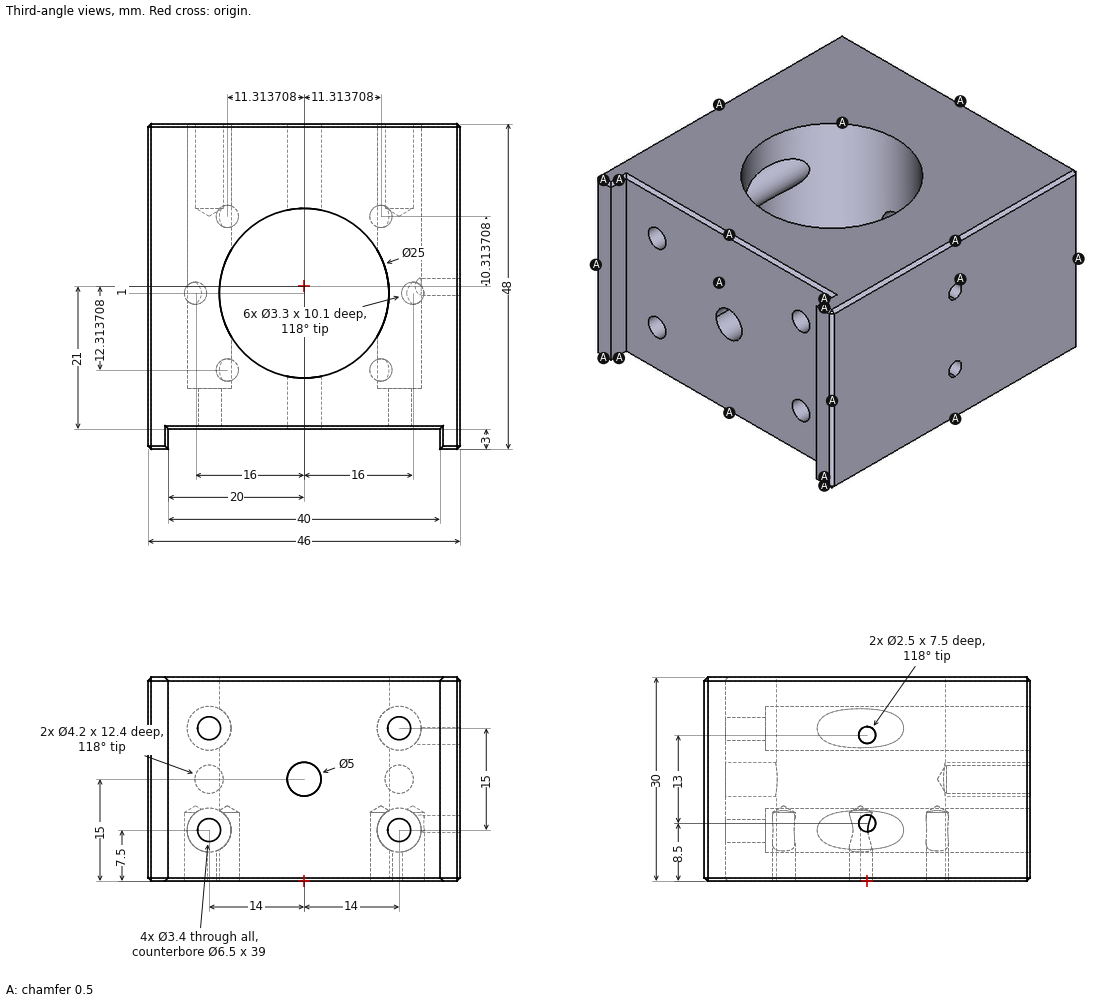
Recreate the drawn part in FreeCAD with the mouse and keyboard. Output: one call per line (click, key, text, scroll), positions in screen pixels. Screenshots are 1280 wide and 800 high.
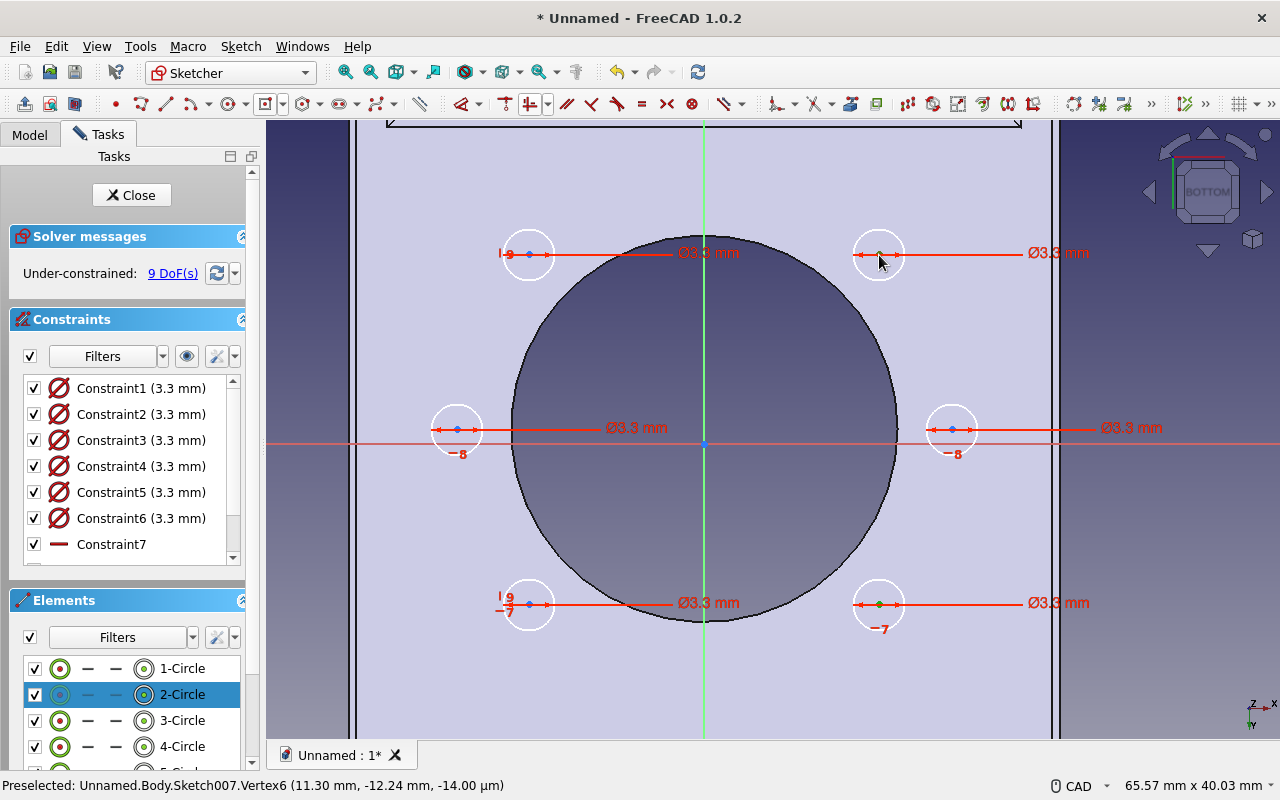
key(v)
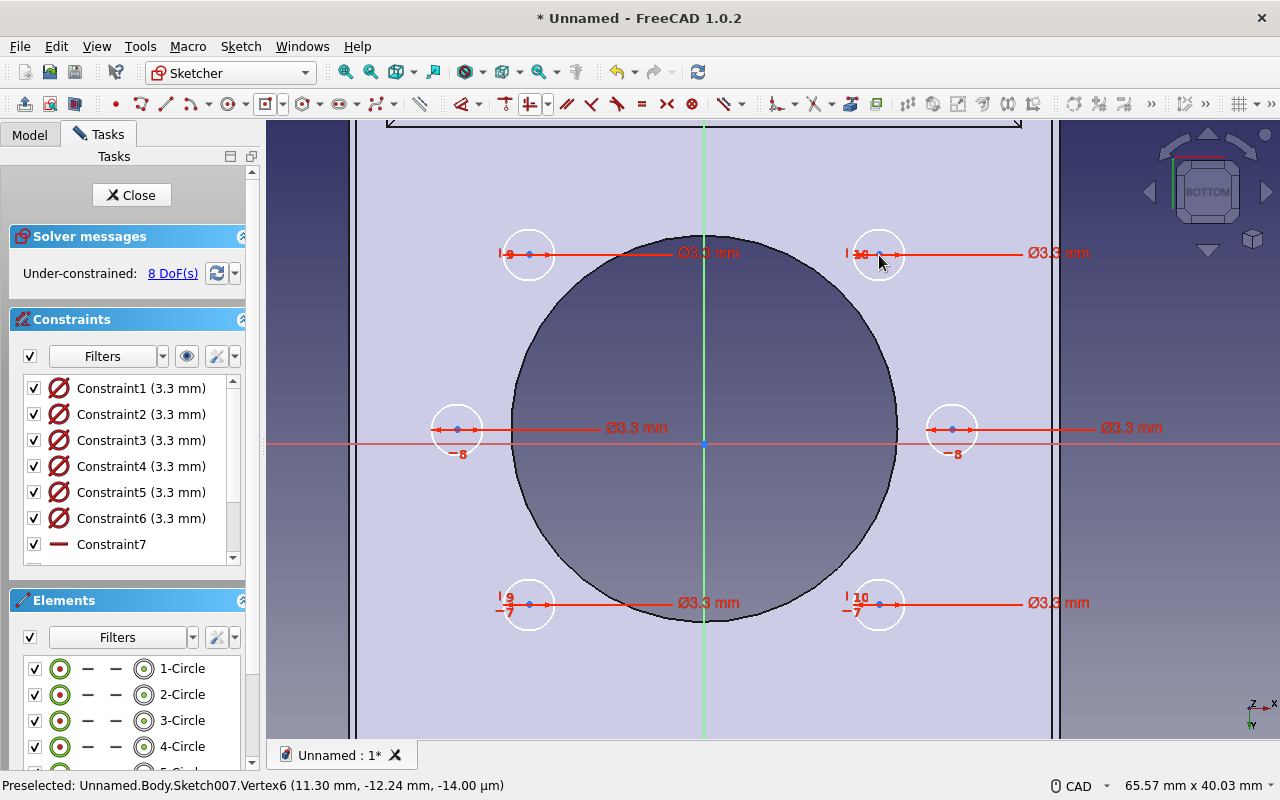
click(529, 255)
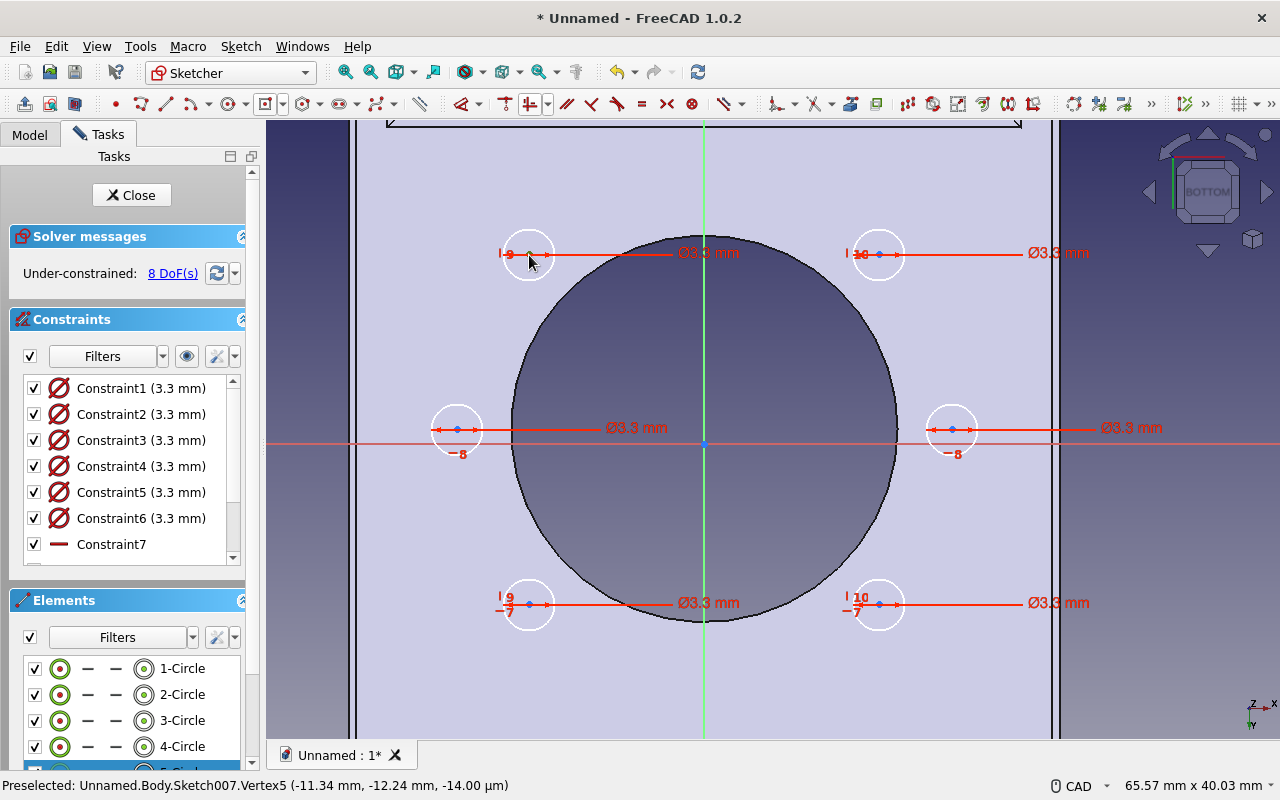
click(879, 255)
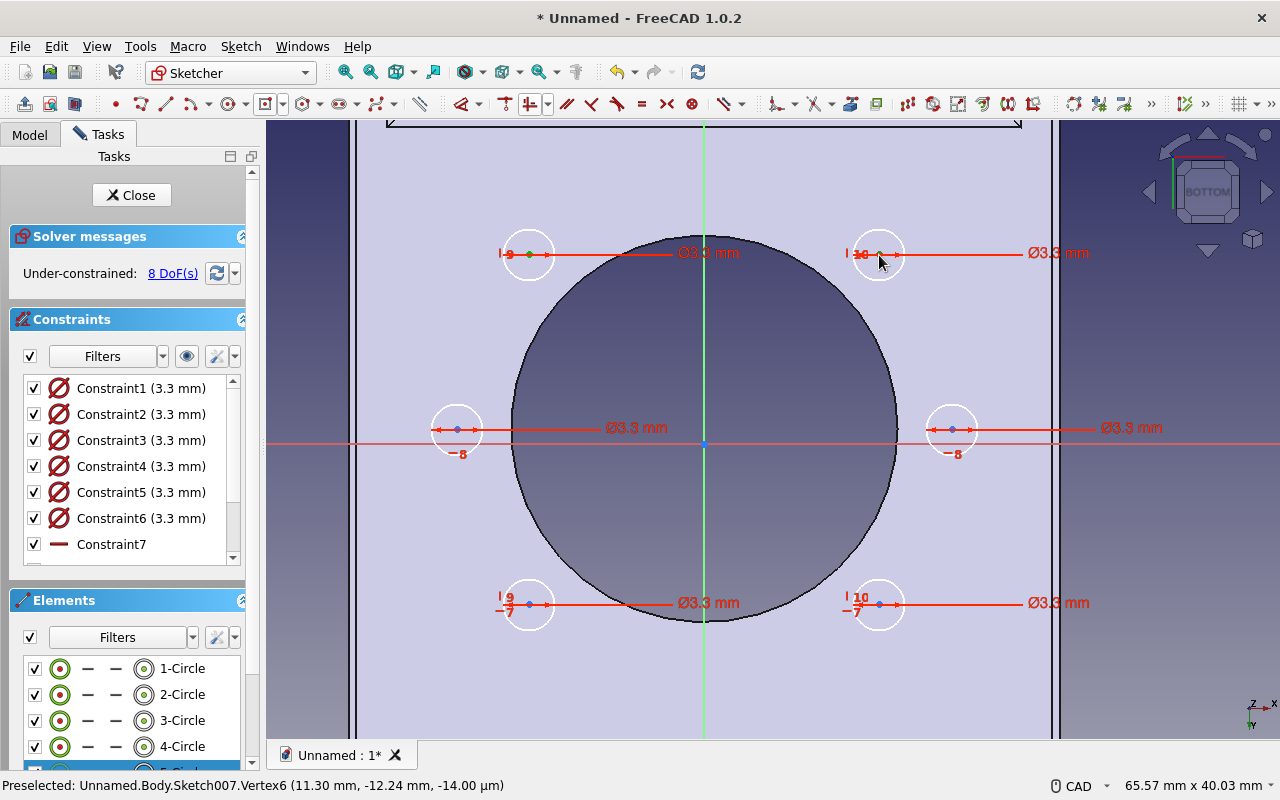
click(548, 104)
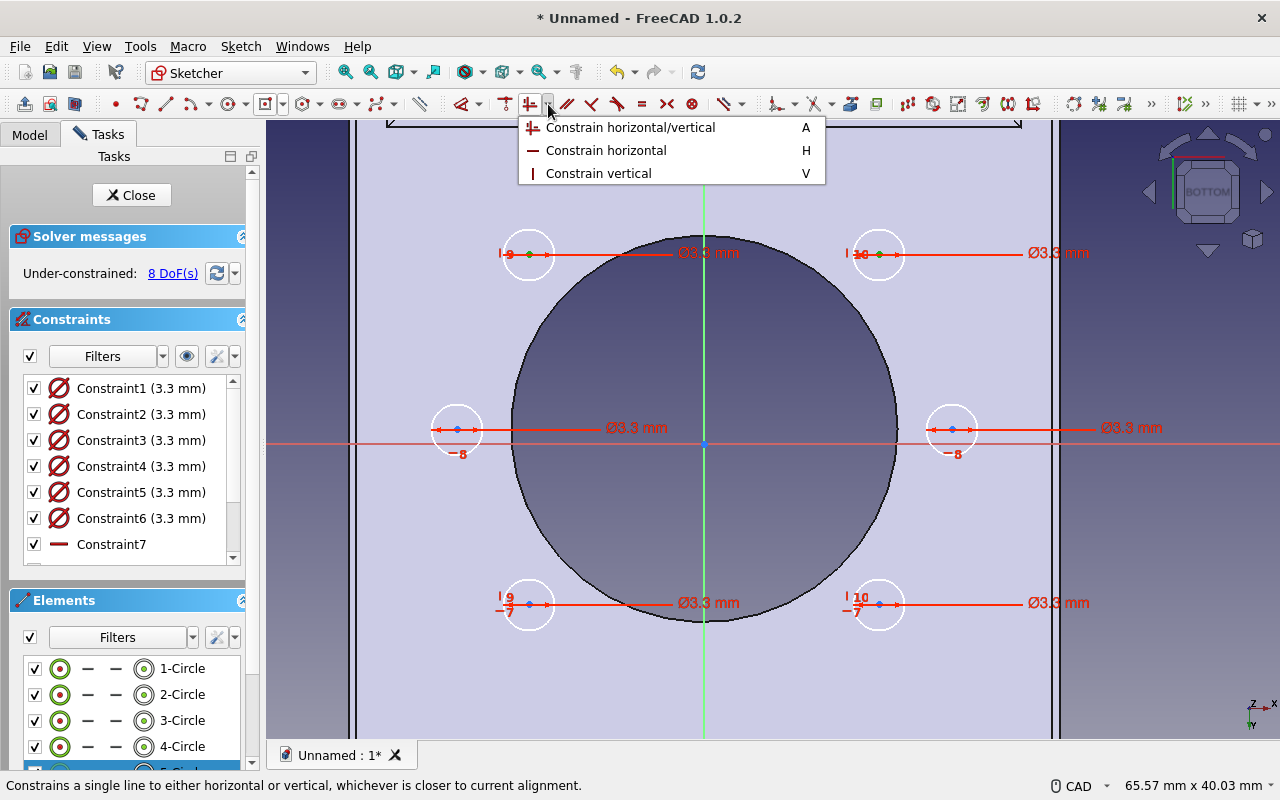
click(672, 150)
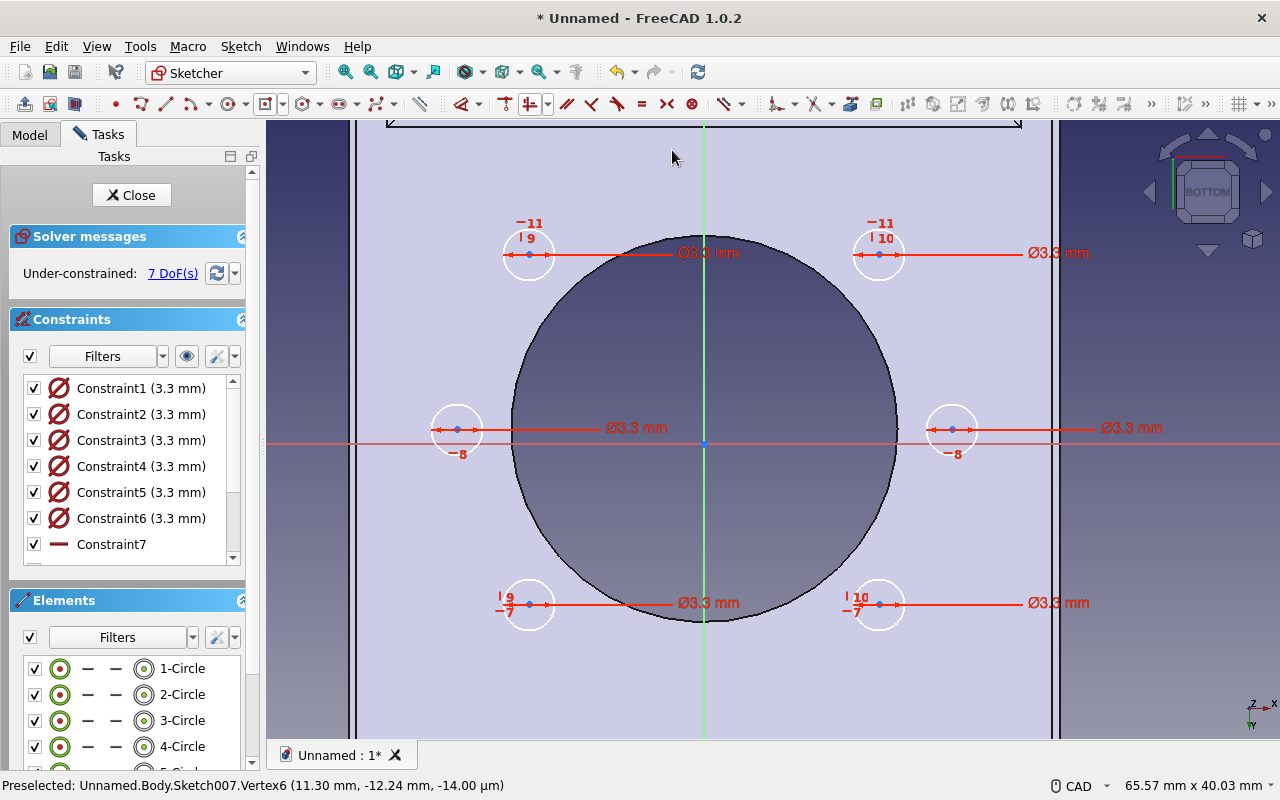
click(460, 104)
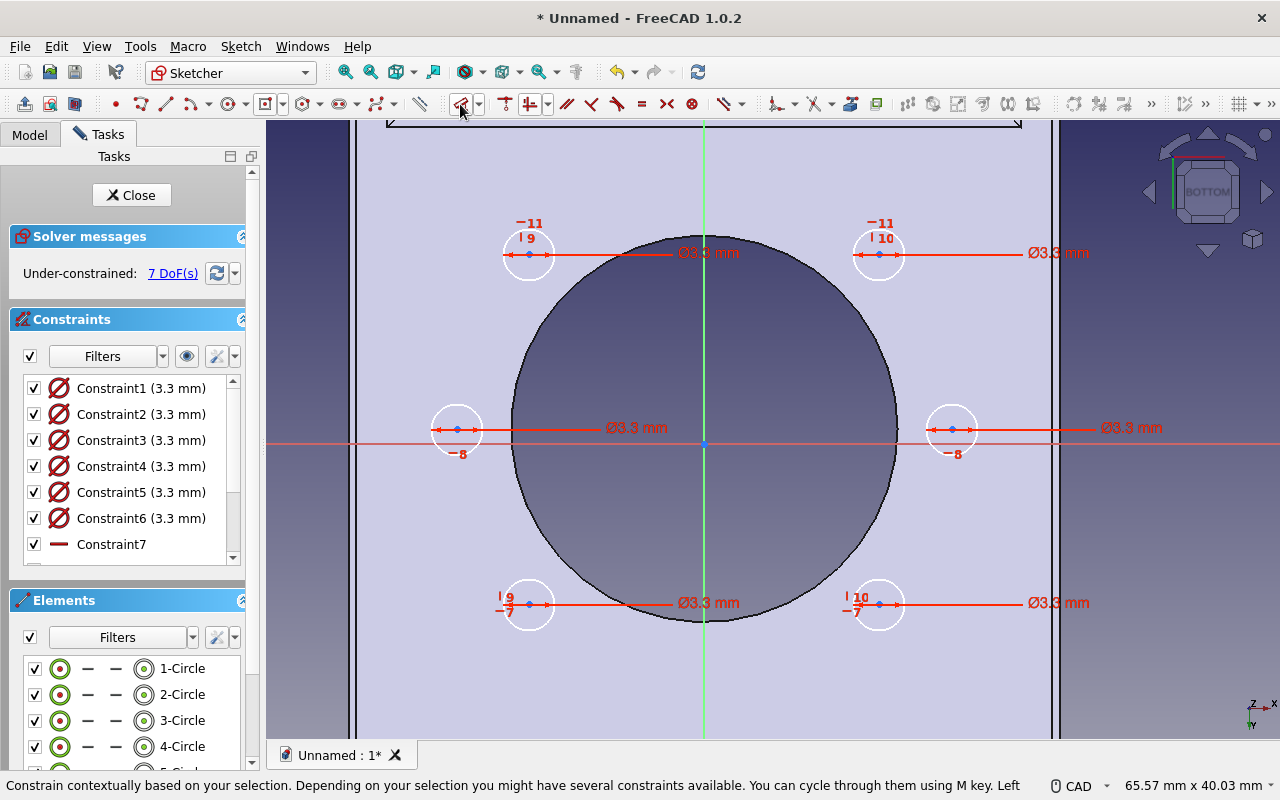
scroll(952, 430, up, 5)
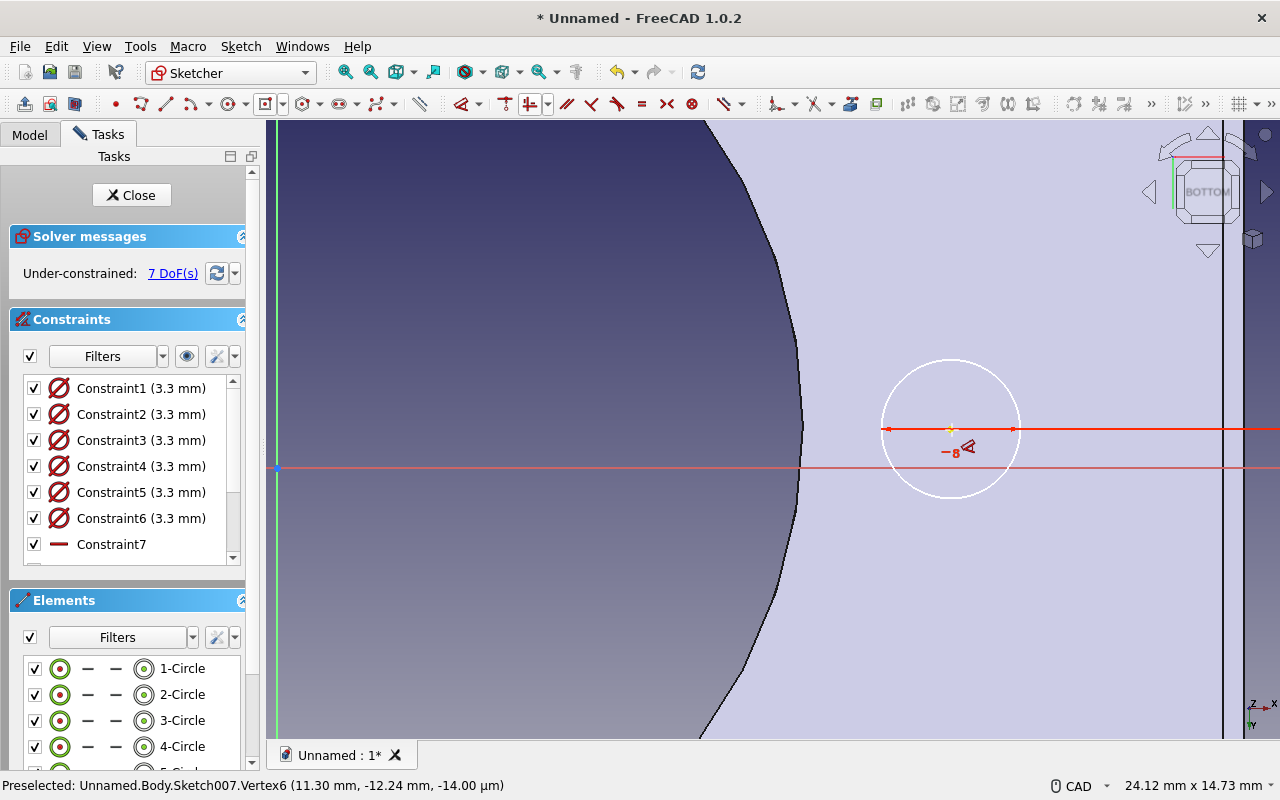
click(951, 429)
click(985, 449)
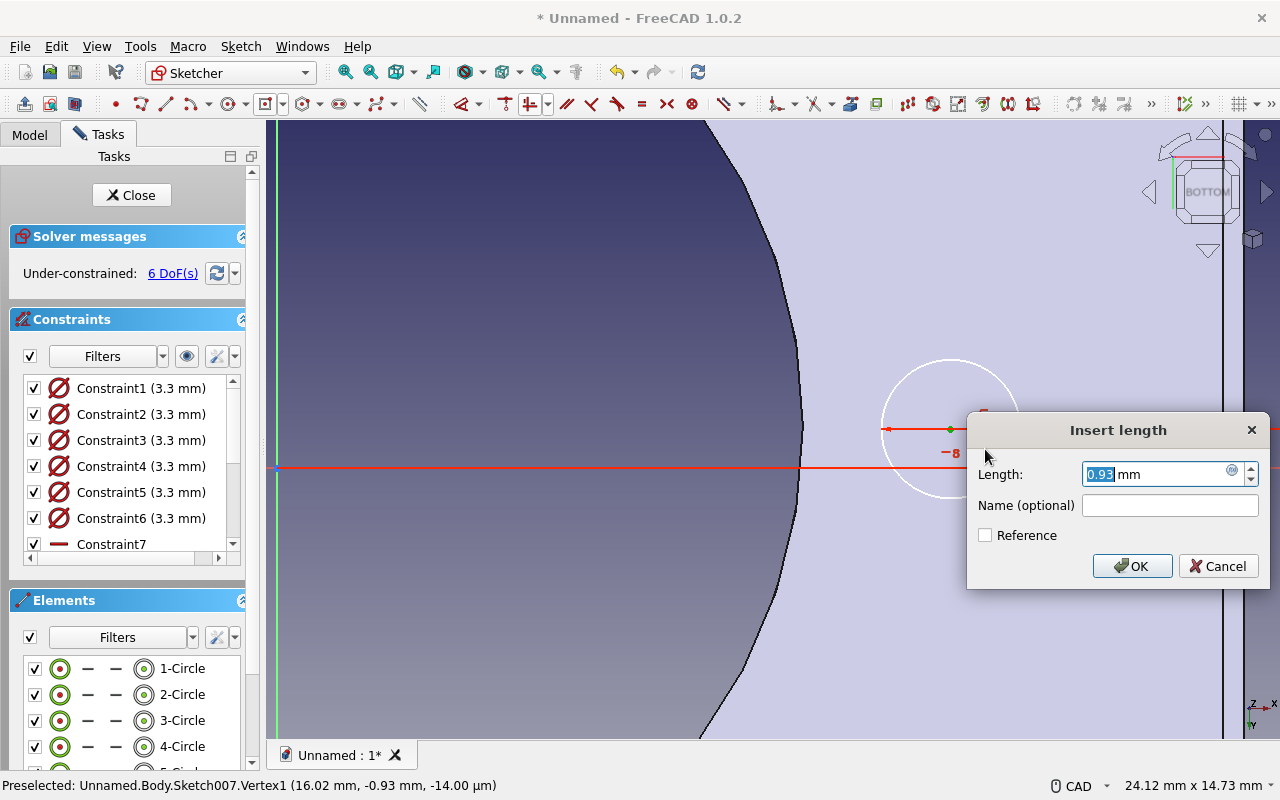
text(1)
key(Return)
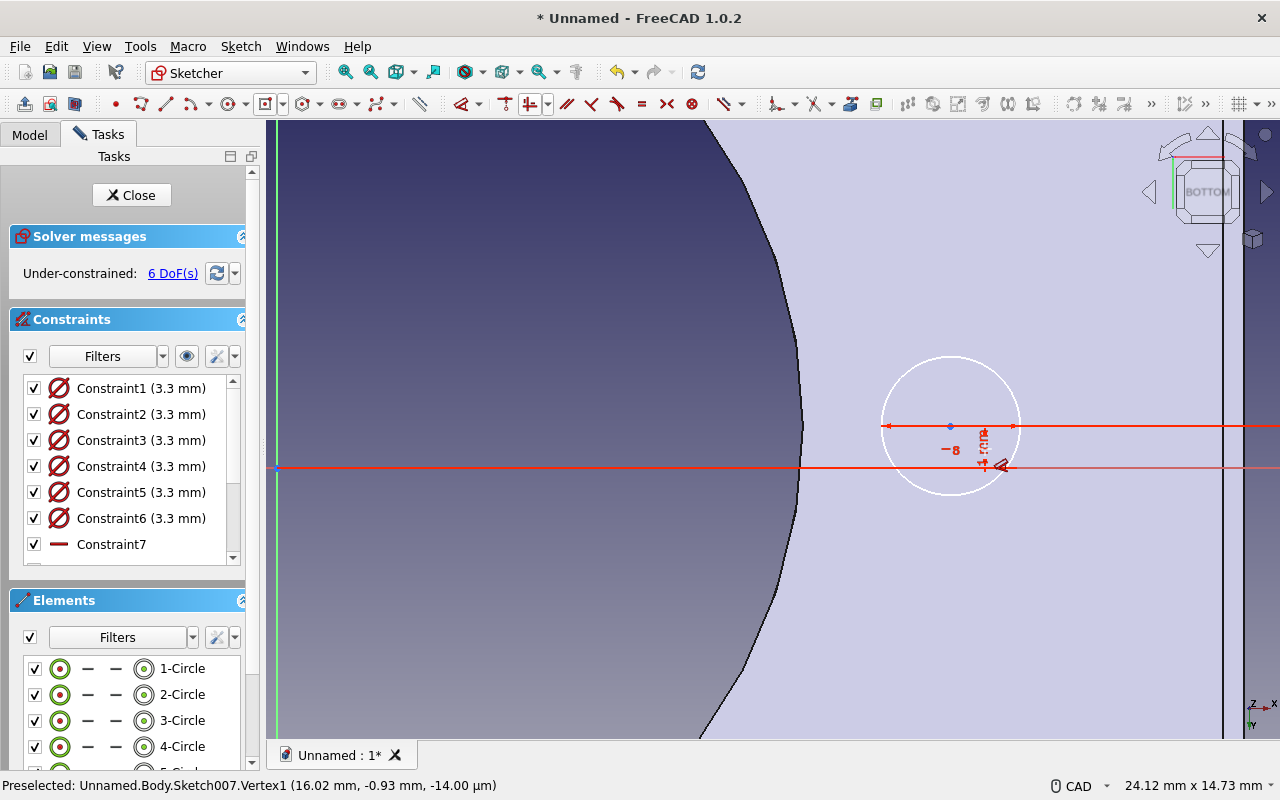
click(951, 426)
click(622, 502)